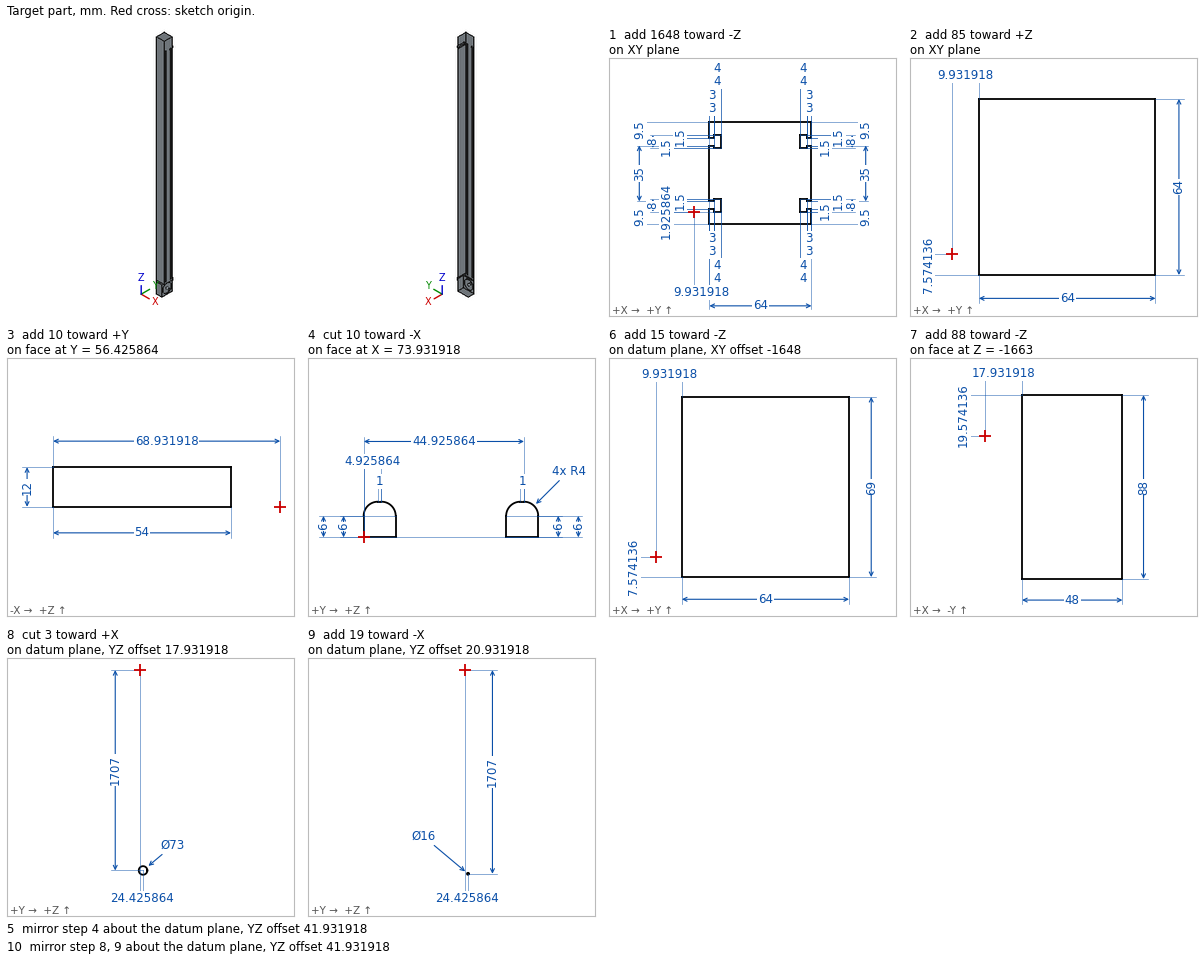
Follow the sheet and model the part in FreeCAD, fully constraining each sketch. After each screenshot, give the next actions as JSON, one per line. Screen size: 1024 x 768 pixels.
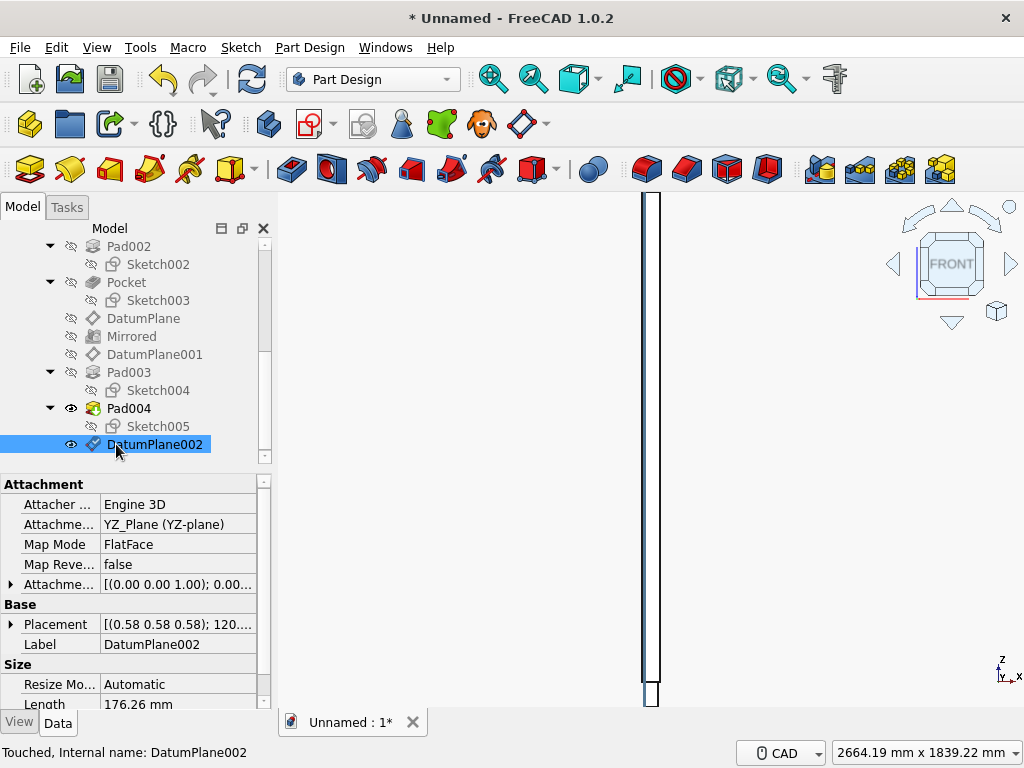
{"action": "left_click", "coordinate": [310, 124]}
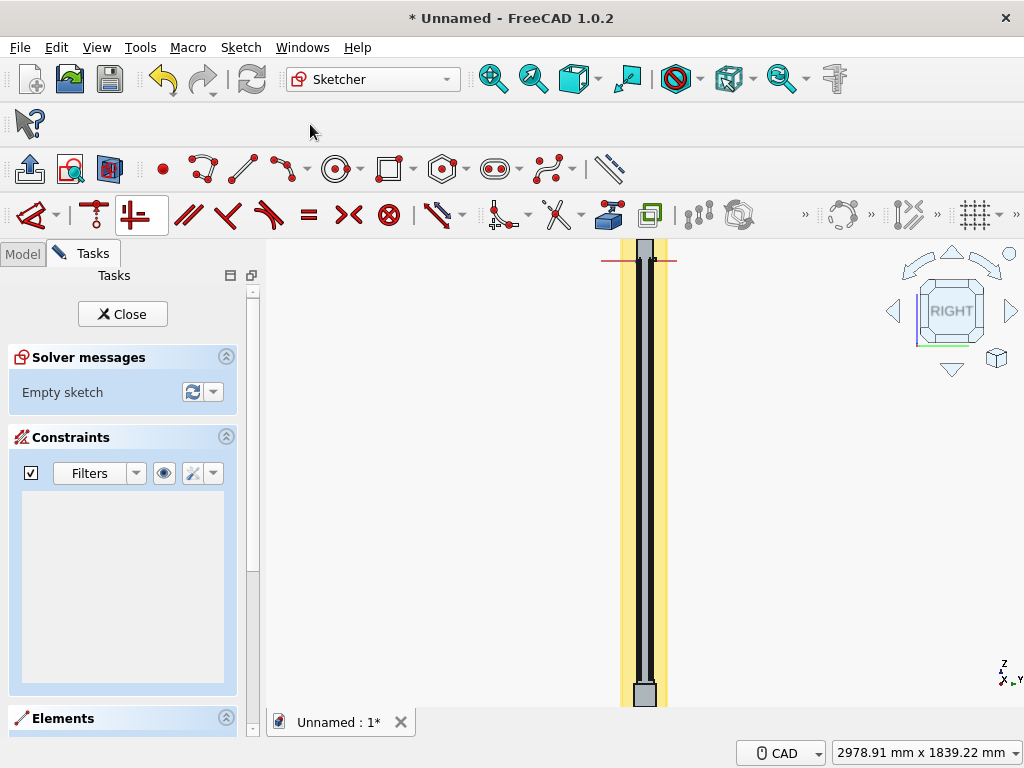
{"action": "left_click", "coordinate": [110, 170]}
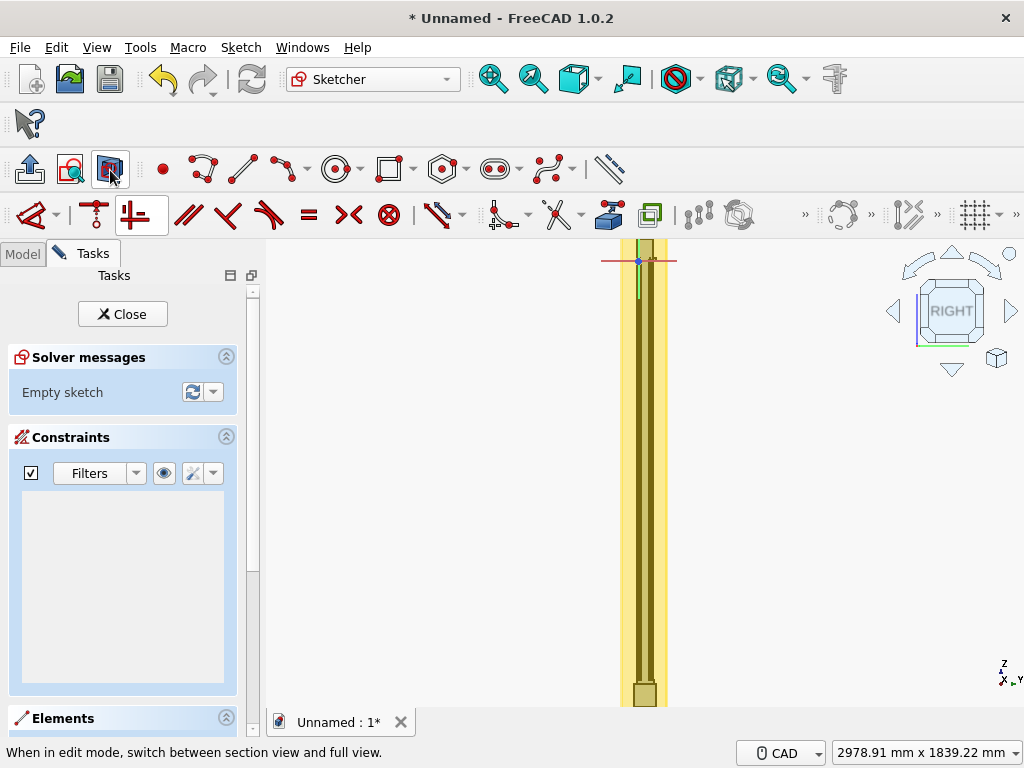
{"action": "scroll", "coordinate": [576, 473], "scroll_direction": "down", "scroll_amount": 5}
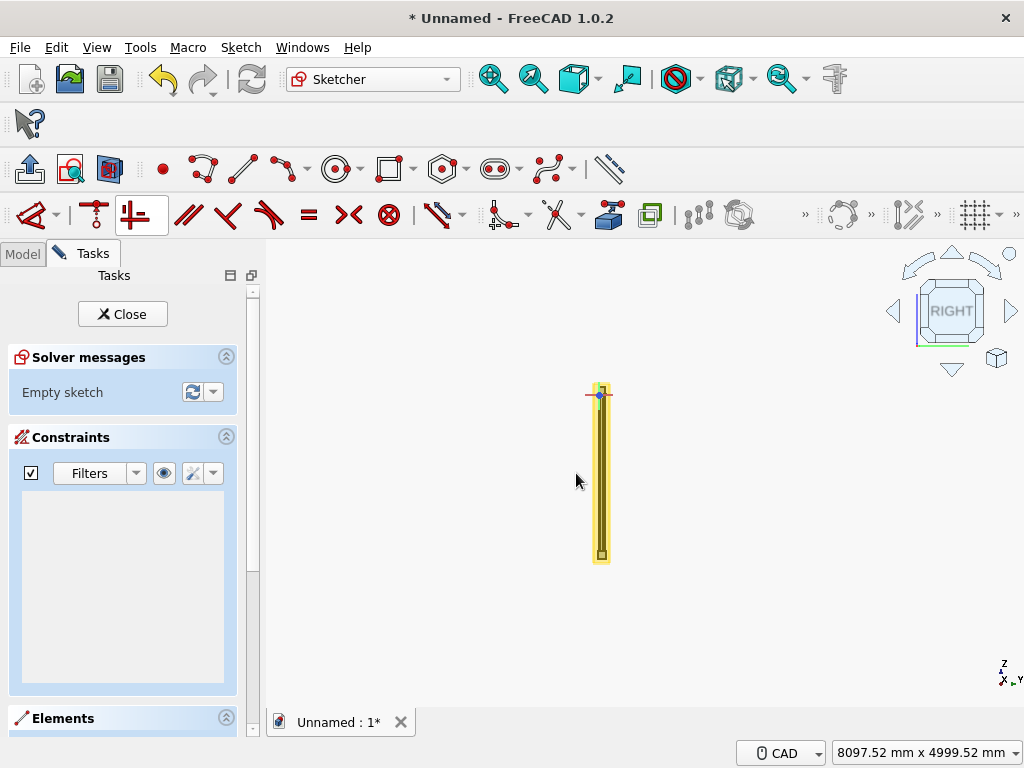
{"action": "scroll", "coordinate": [603, 559], "scroll_direction": "up", "scroll_amount": 15}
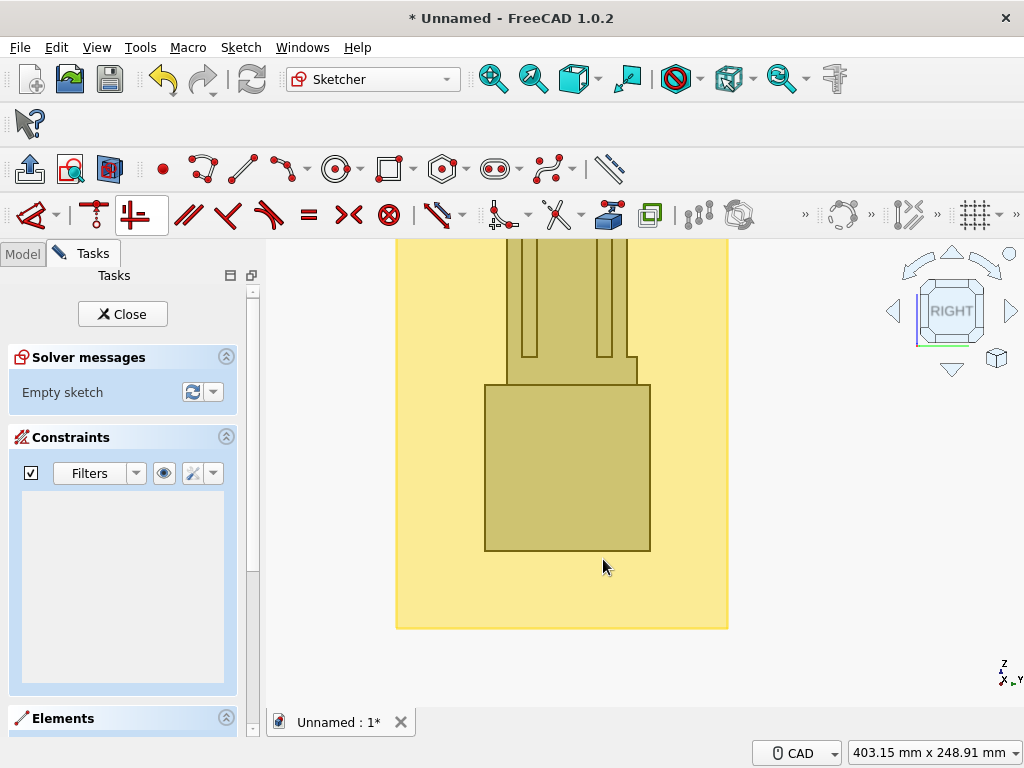
{"action": "scroll", "coordinate": [560, 464], "scroll_direction": "up", "scroll_amount": 4}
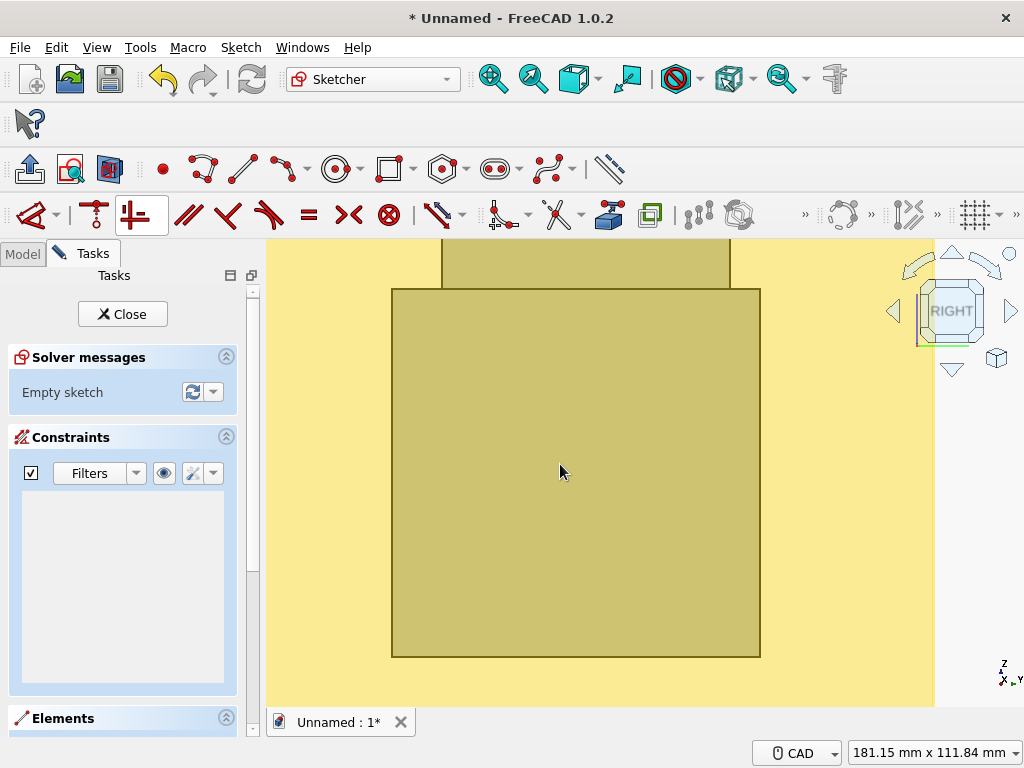
{"action": "left_click", "coordinate": [336, 170]}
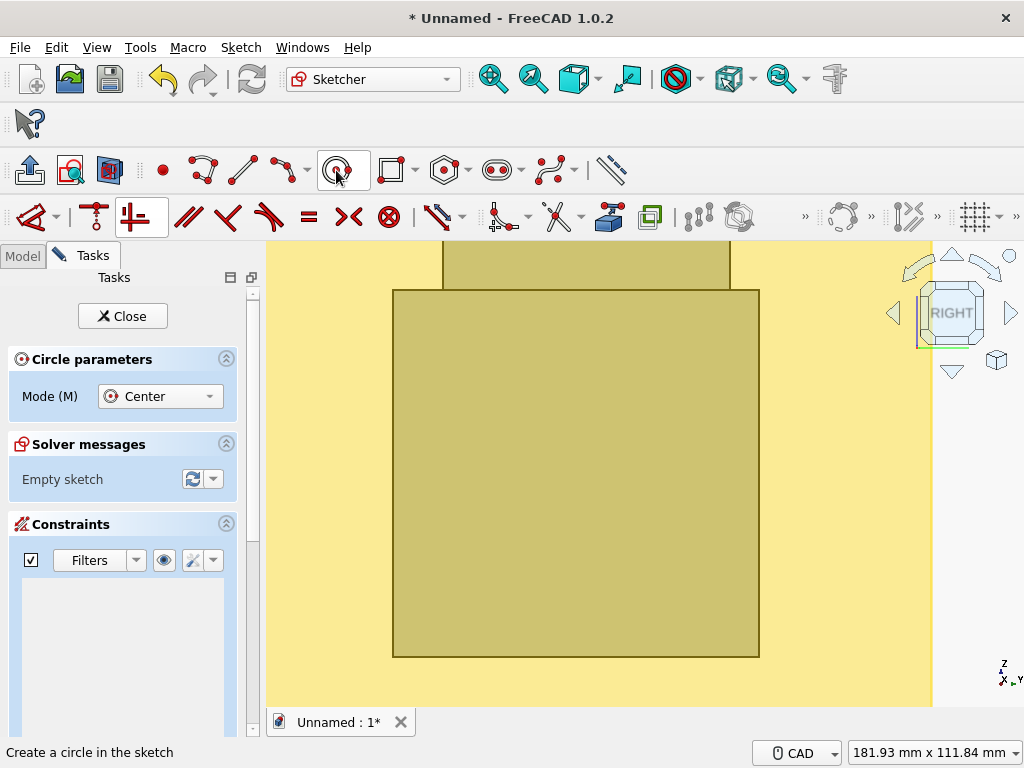
{"action": "left_click", "coordinate": [576, 474]}
{"action": "mouse_move", "coordinate": [683, 366]}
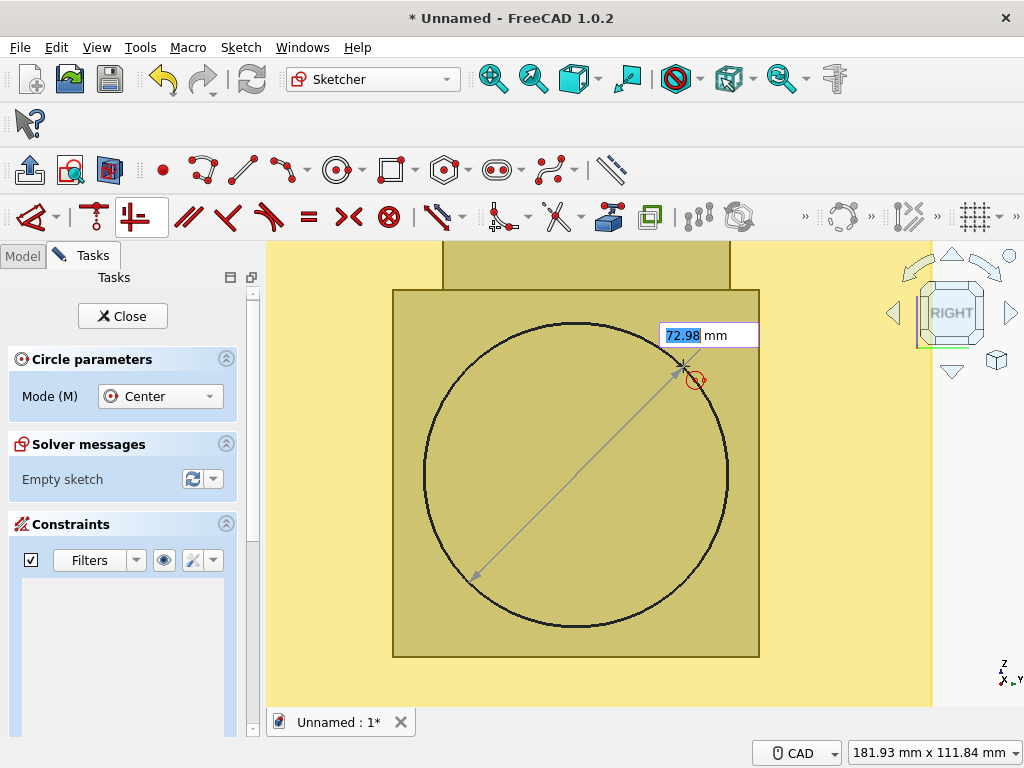
{"action": "type", "text": "73"}
{"action": "key", "text": "Return"}
{"action": "key", "text": "Escape"}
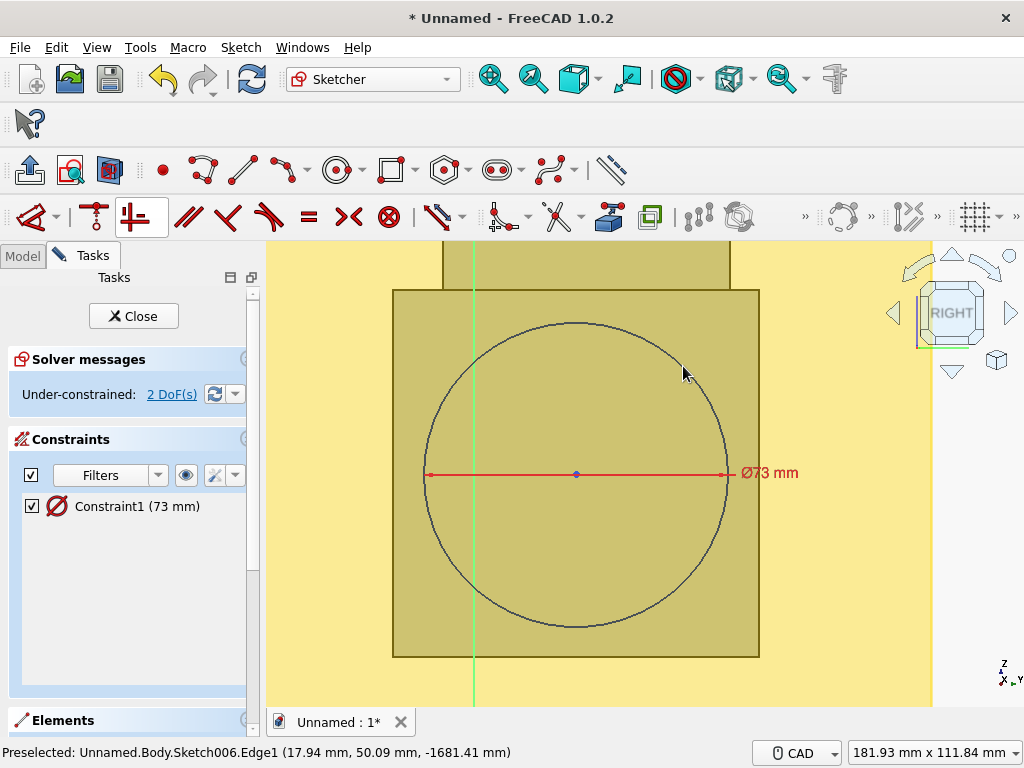
{"action": "left_click", "coordinate": [32, 218]}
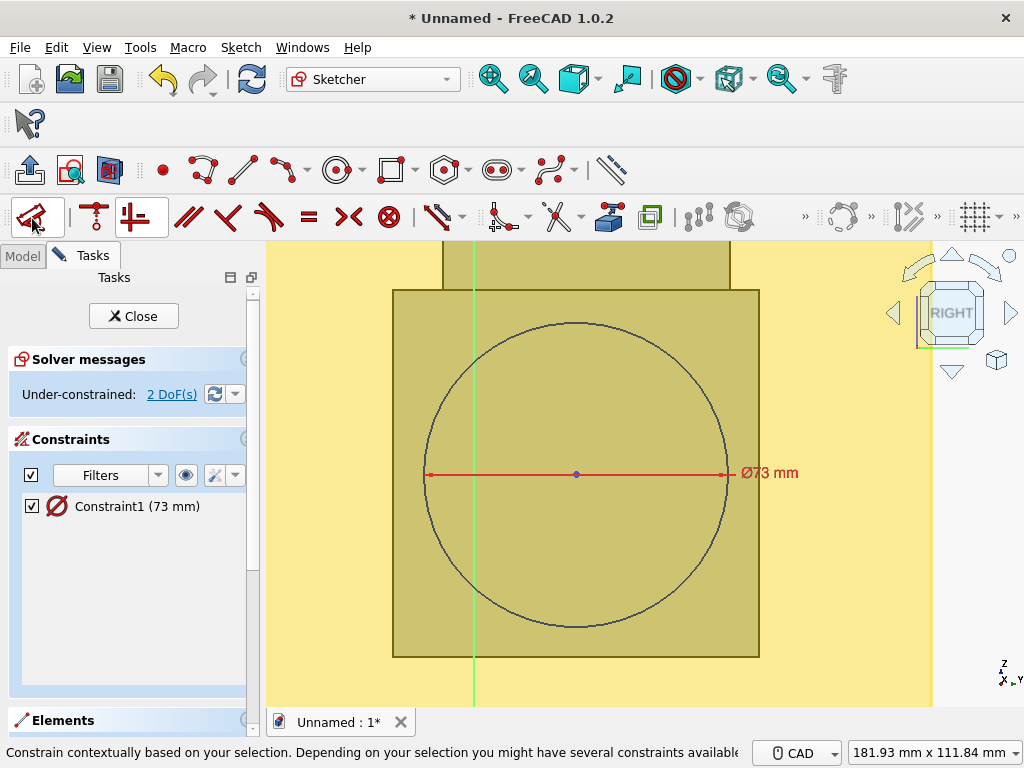
{"action": "left_click", "coordinate": [576, 475]}
{"action": "left_click", "coordinate": [440, 372]}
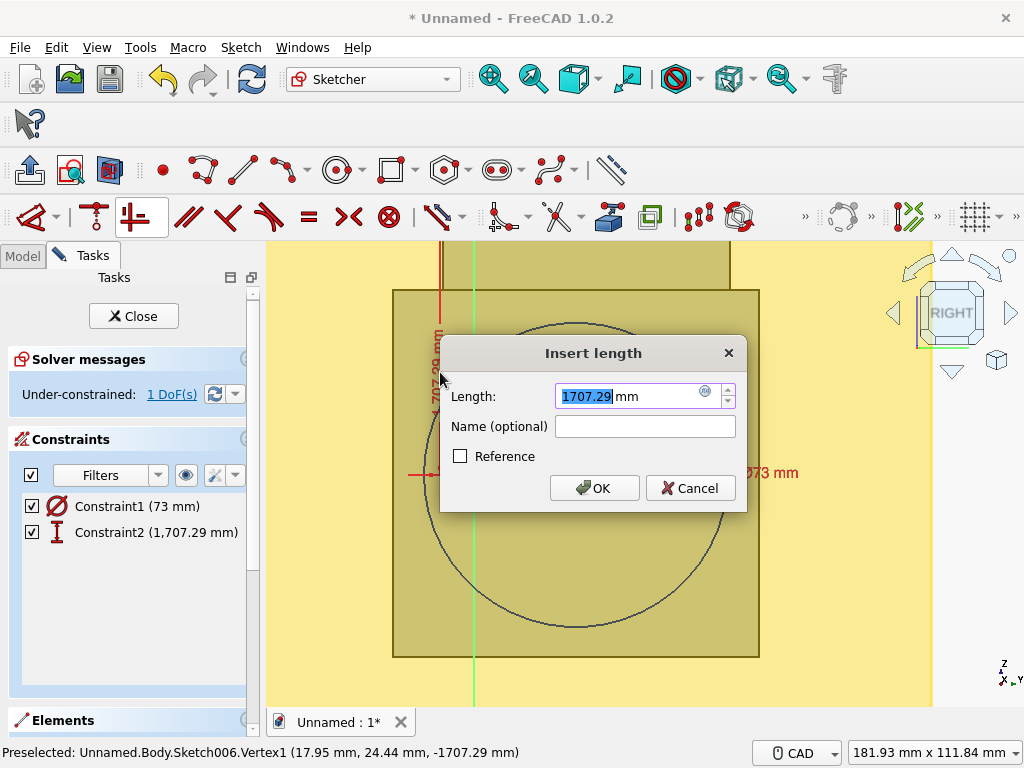
{"action": "type", "text": "1707"}
{"action": "key", "text": "Return"}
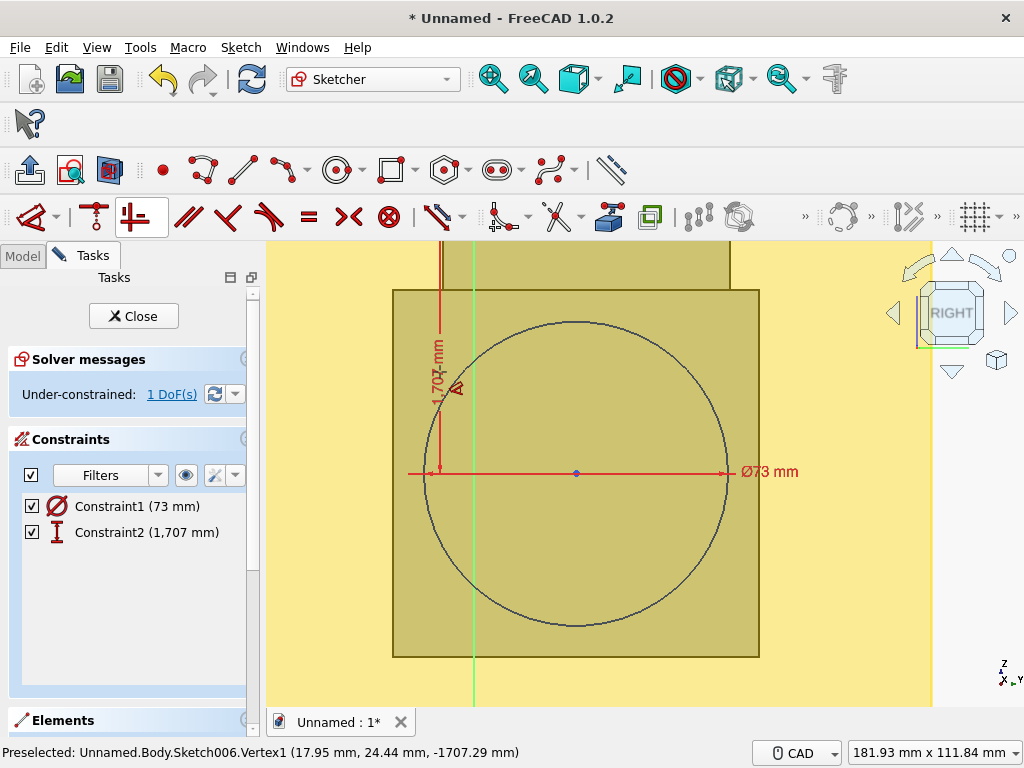
{"action": "left_click", "coordinate": [576, 474]}
{"action": "left_click", "coordinate": [525, 508]}